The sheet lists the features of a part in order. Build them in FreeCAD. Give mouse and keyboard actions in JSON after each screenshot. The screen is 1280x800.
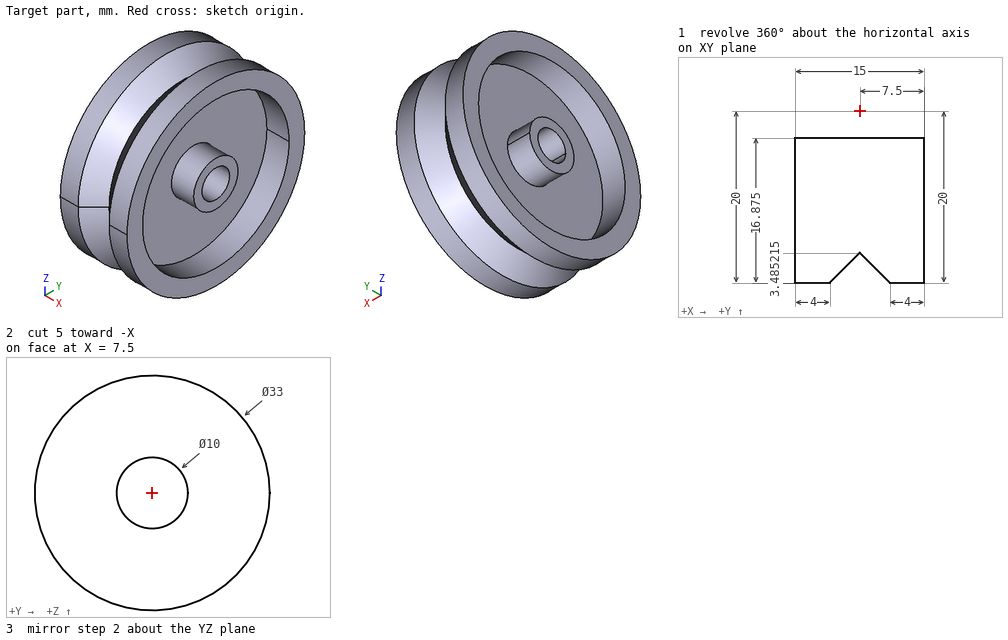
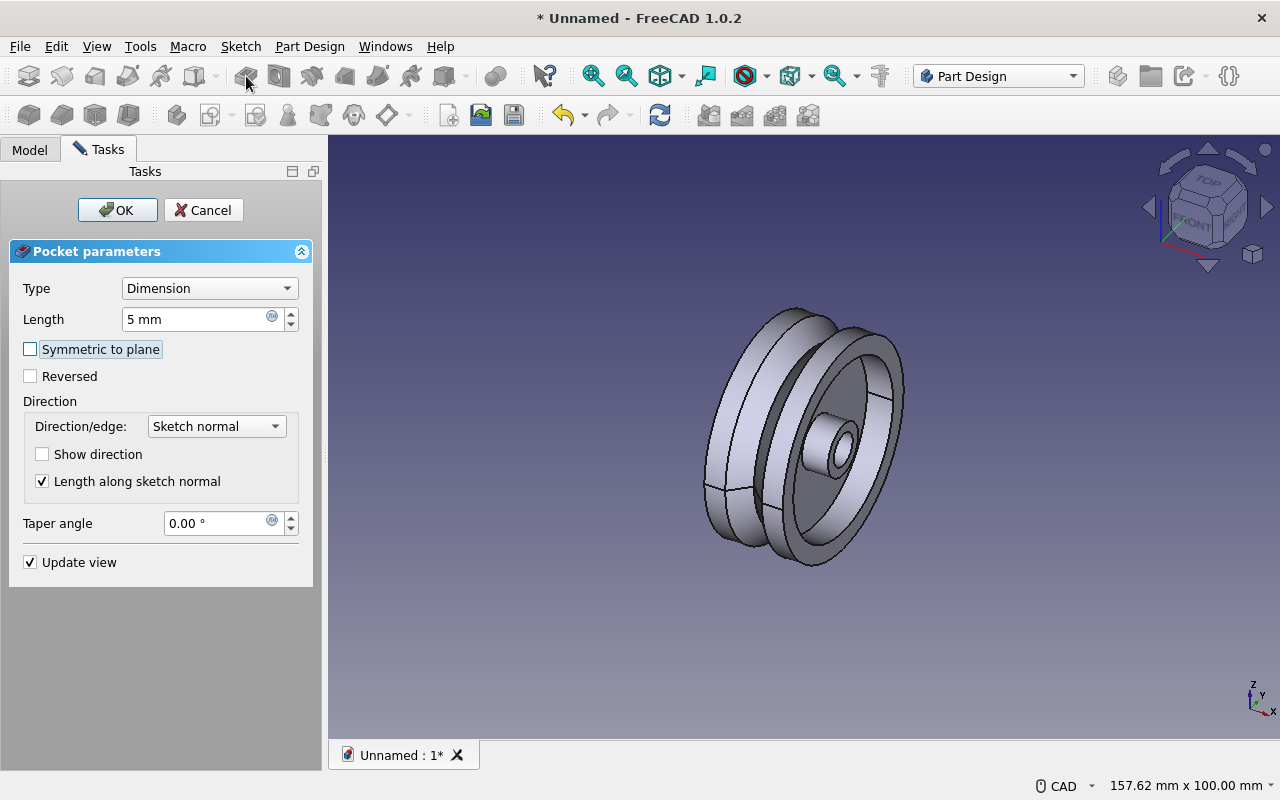
{"action": "left_click", "coordinate": [118, 210]}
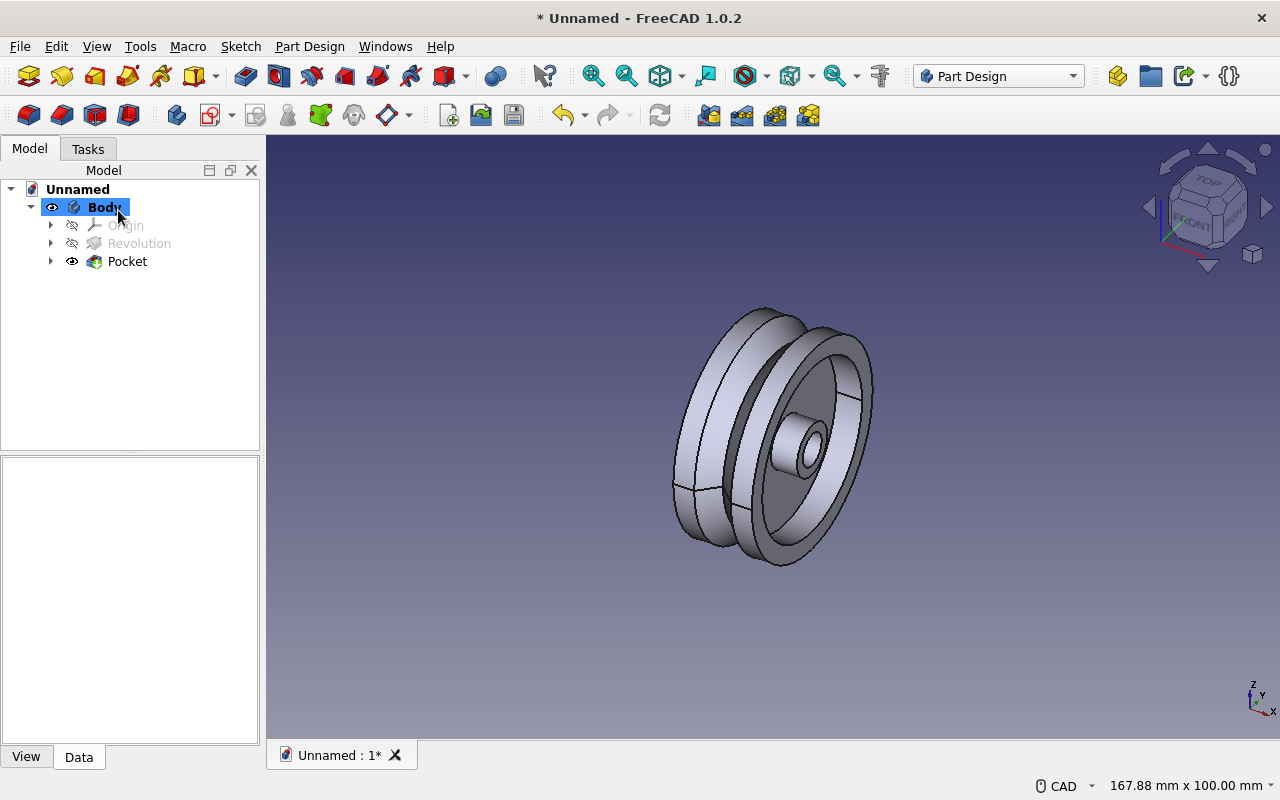
{"action": "left_click", "coordinate": [117, 261]}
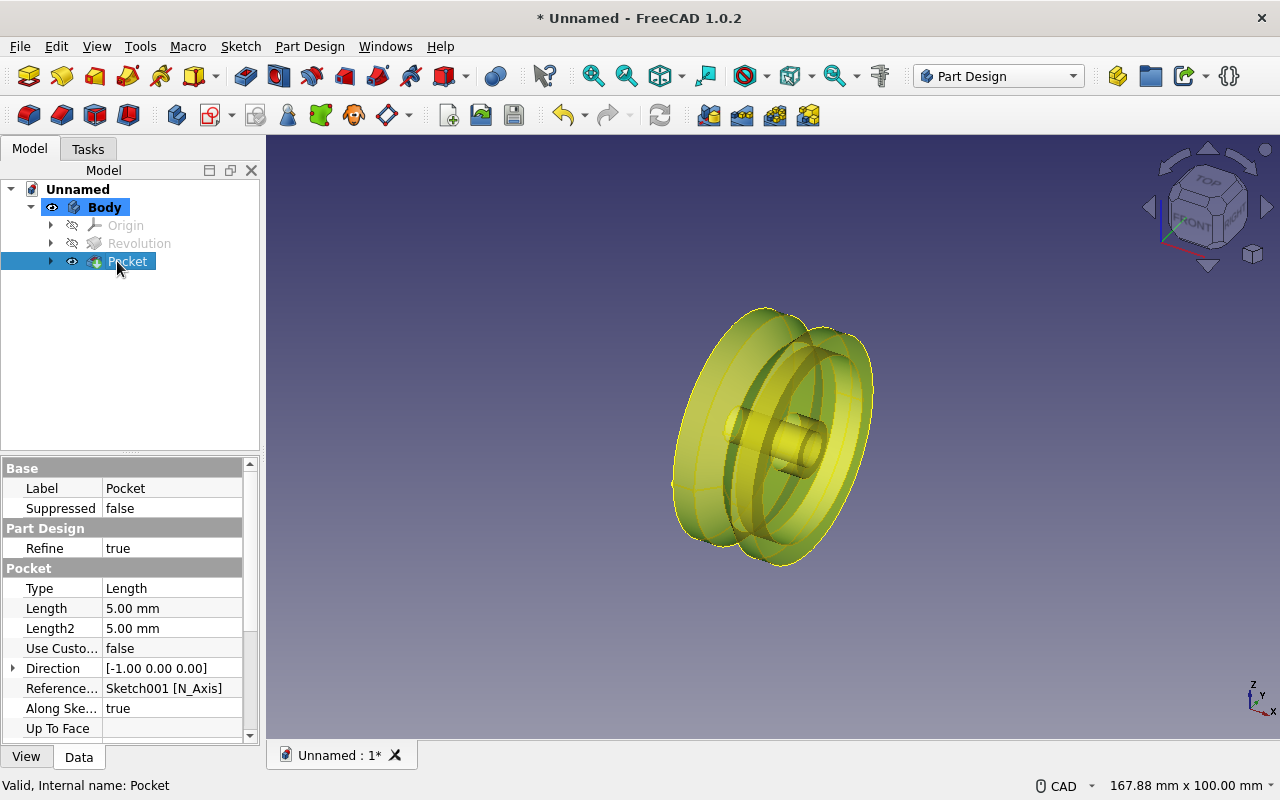
{"action": "left_click", "coordinate": [709, 116]}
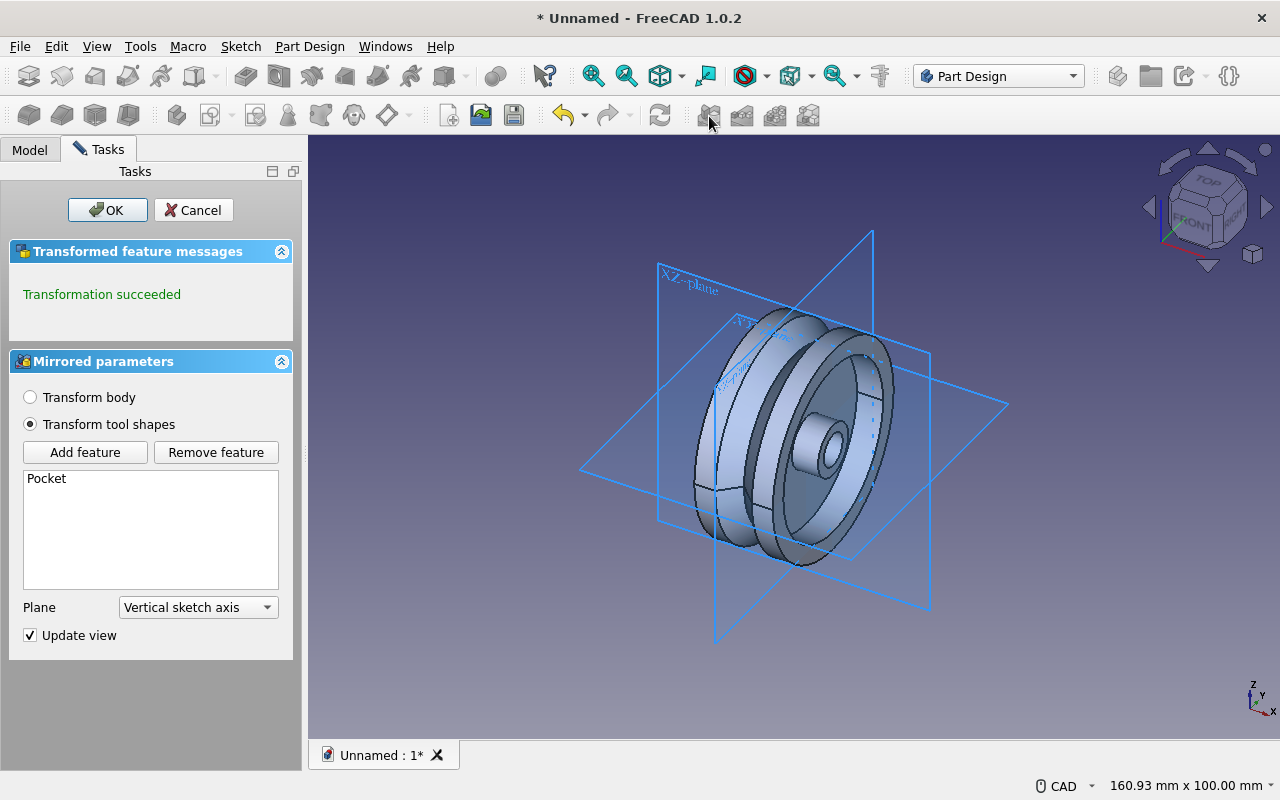
{"action": "left_click", "coordinate": [199, 608]}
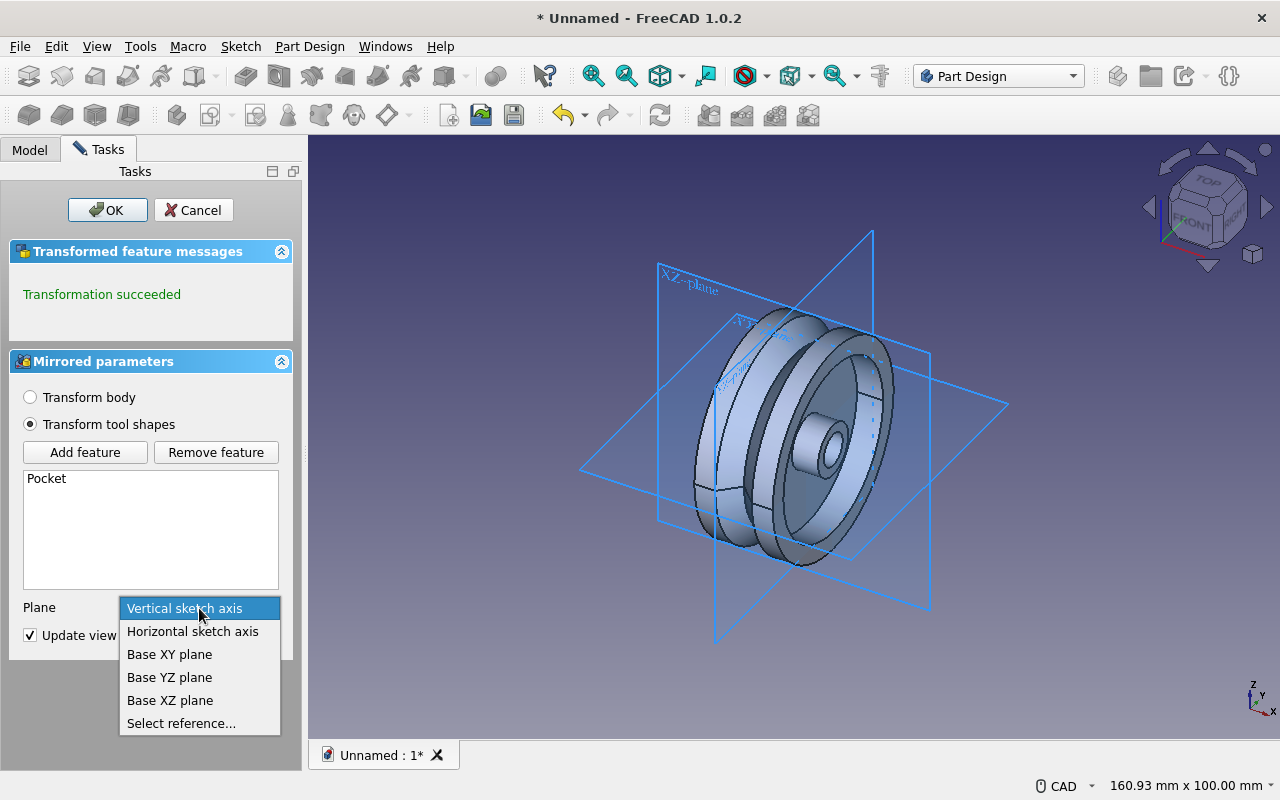
{"action": "left_click", "coordinate": [198, 678]}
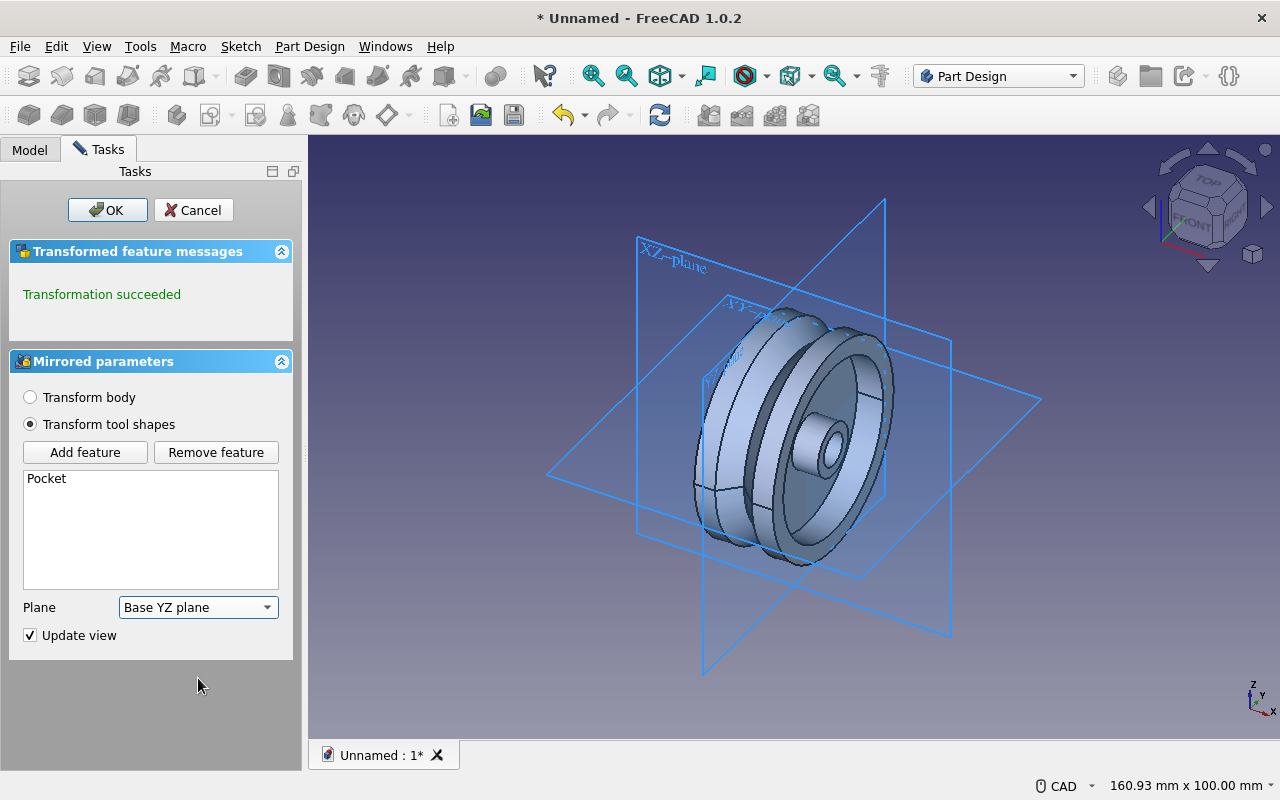
{"action": "left_click", "coordinate": [108, 210]}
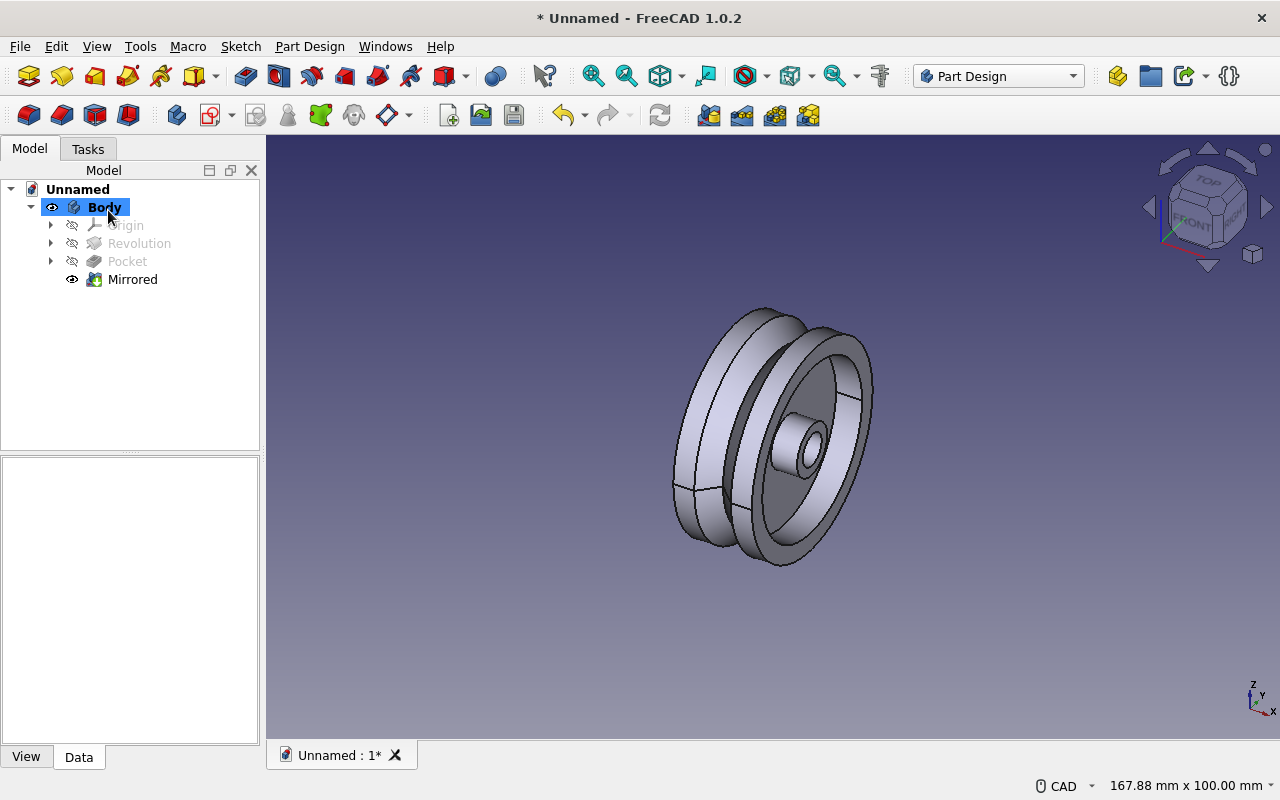
{"action": "key", "text": "0"}